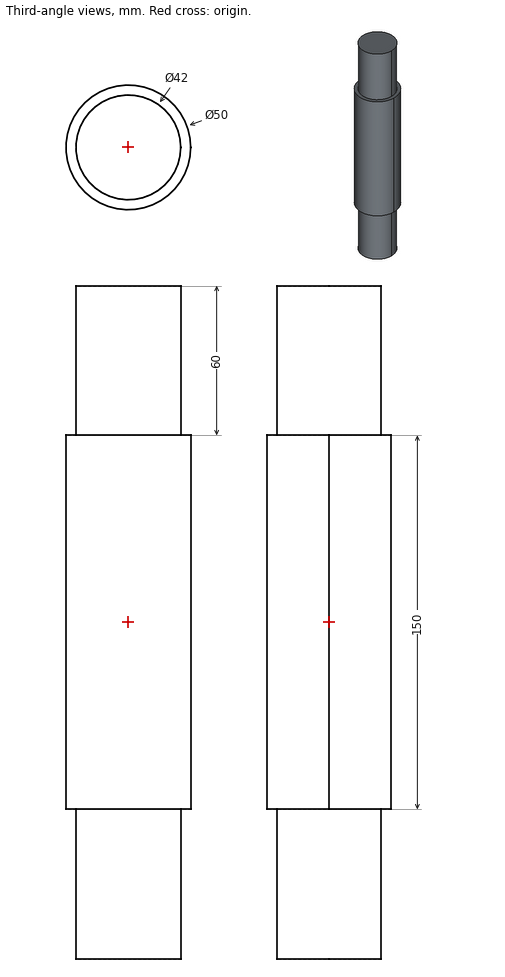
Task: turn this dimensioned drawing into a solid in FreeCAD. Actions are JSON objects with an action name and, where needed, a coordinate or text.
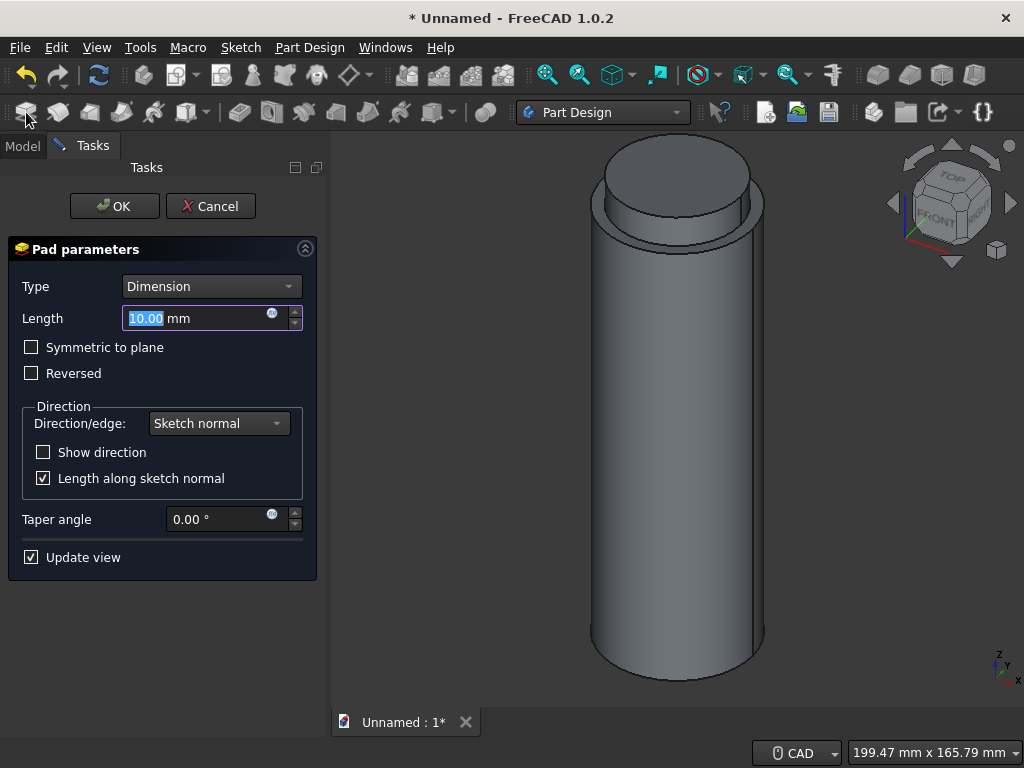
{"action": "type", "text": "60"}
{"action": "key", "text": "Tab"}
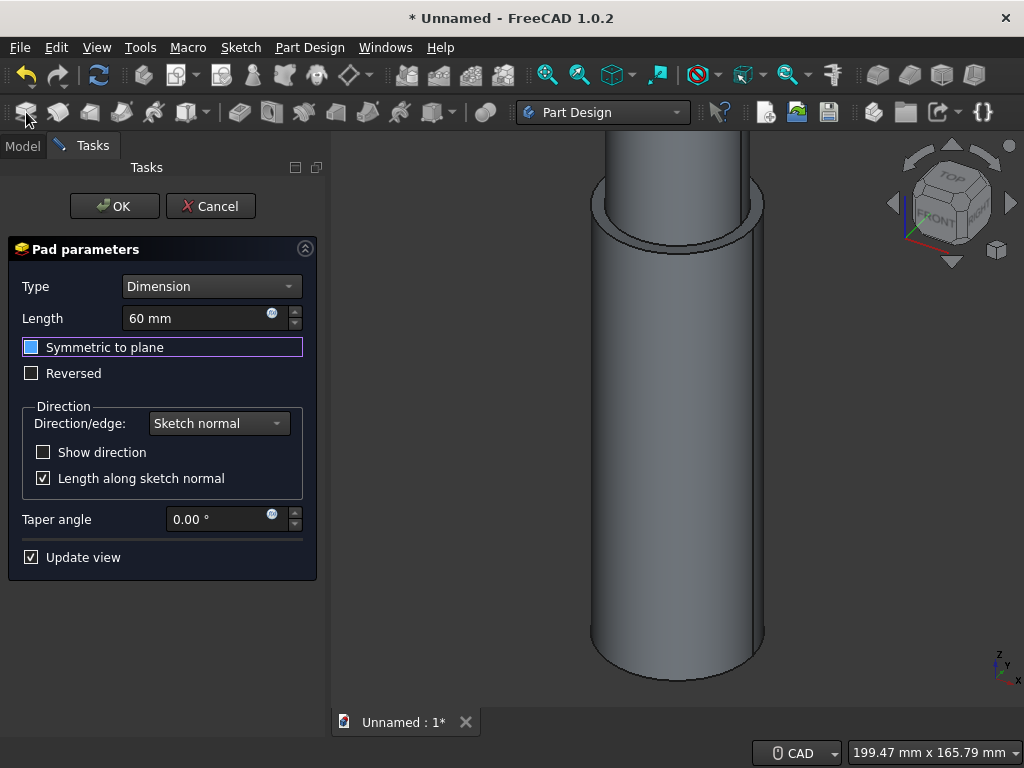
{"action": "left_click", "coordinate": [115, 206]}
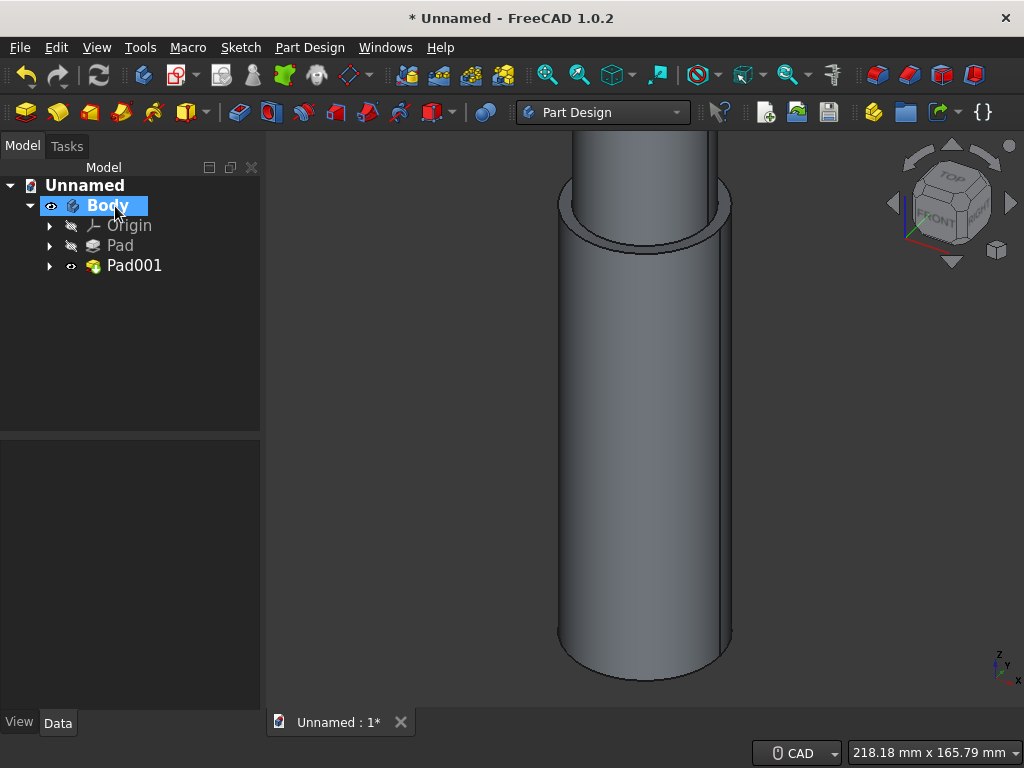
{"action": "left_click", "coordinate": [548, 76]}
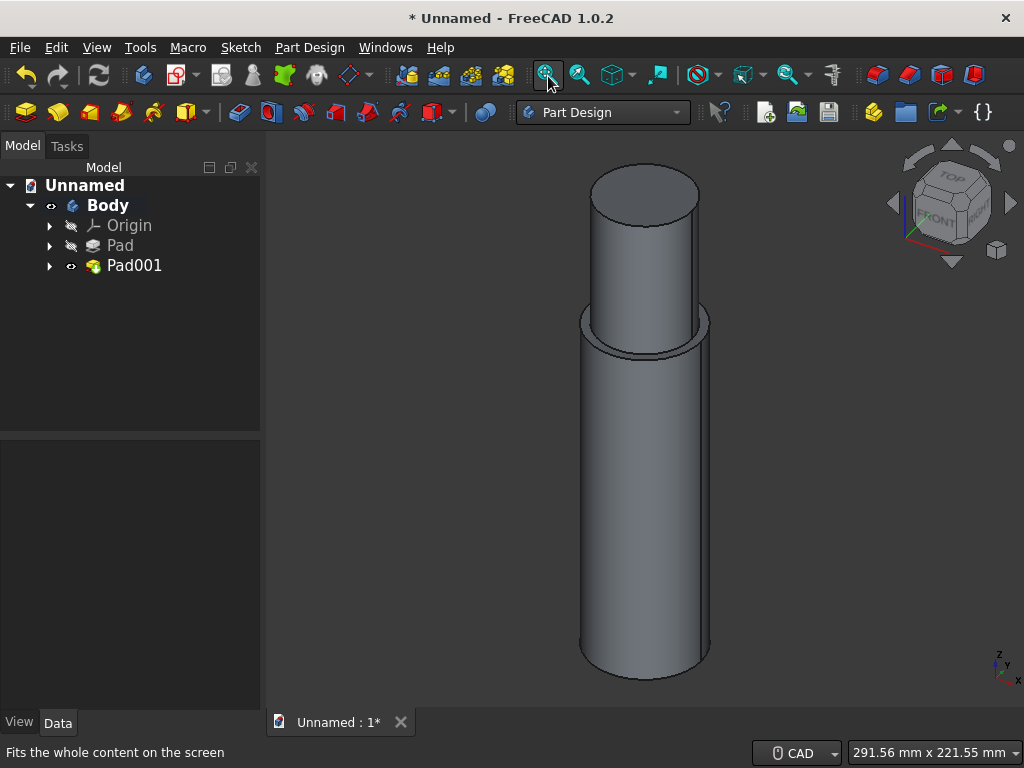
{"action": "left_click", "coordinate": [116, 266]}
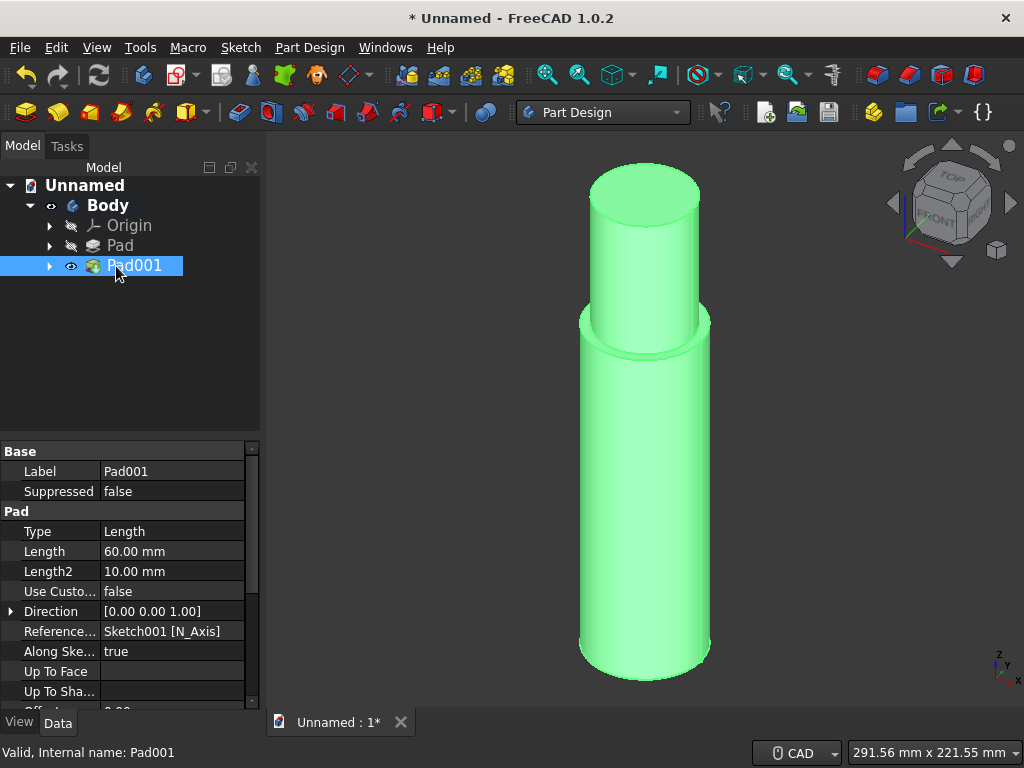
{"action": "left_click", "coordinate": [408, 76]}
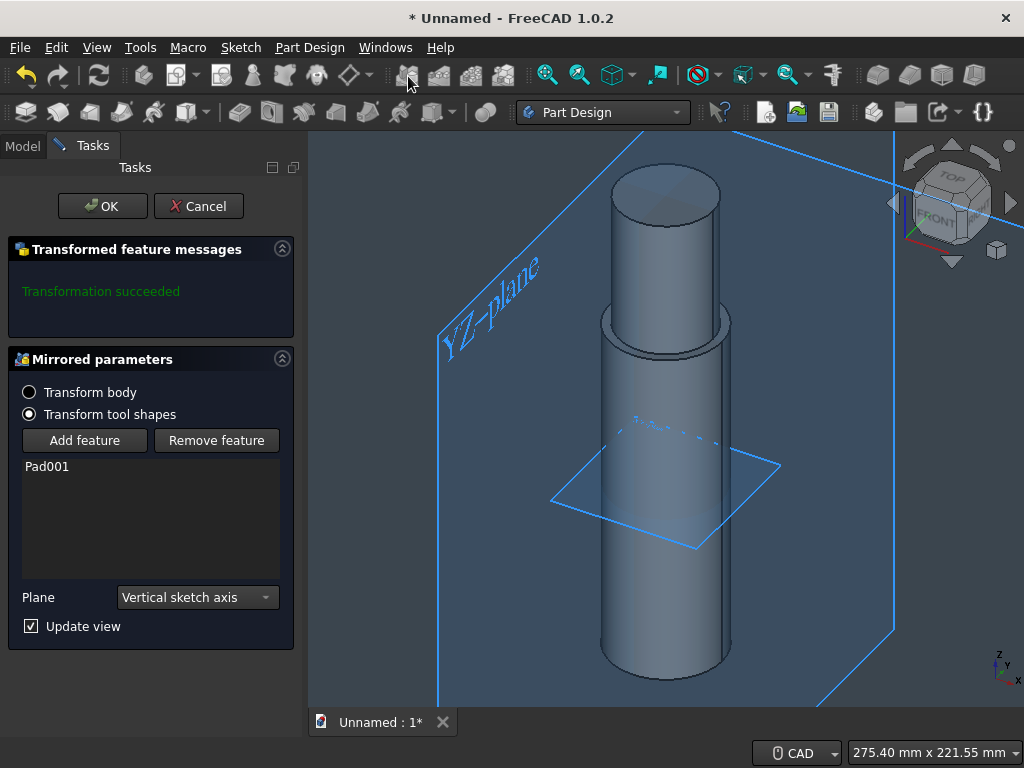
{"action": "left_click", "coordinate": [198, 598]}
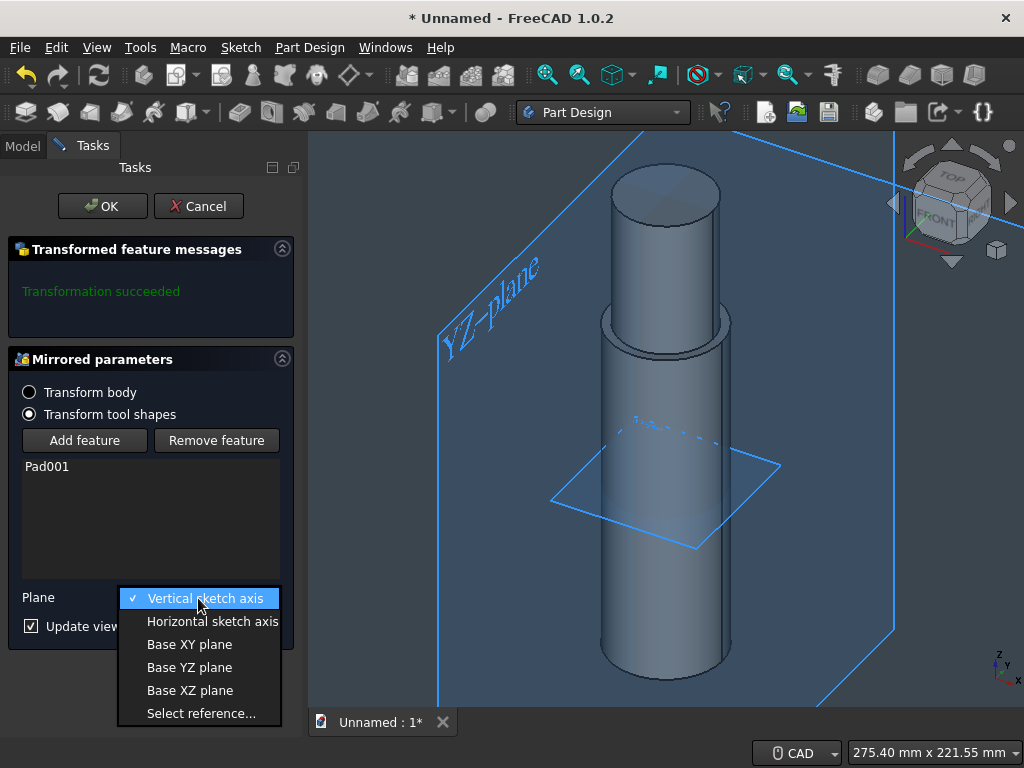
{"action": "left_click", "coordinate": [198, 644]}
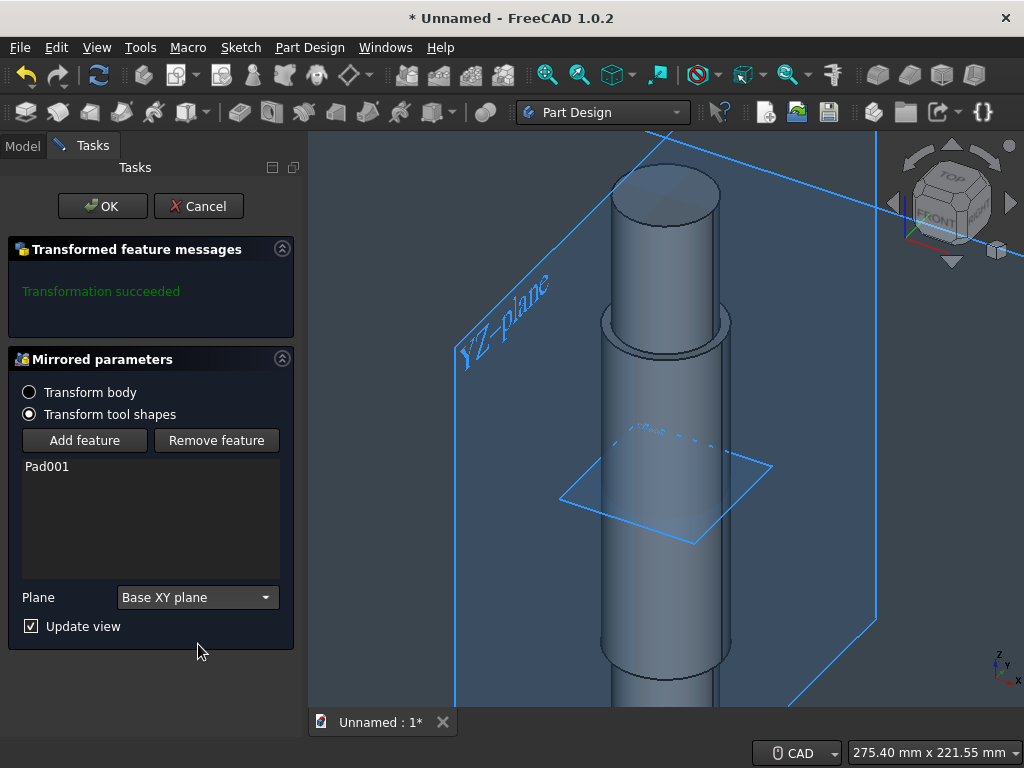
{"action": "left_click", "coordinate": [103, 206]}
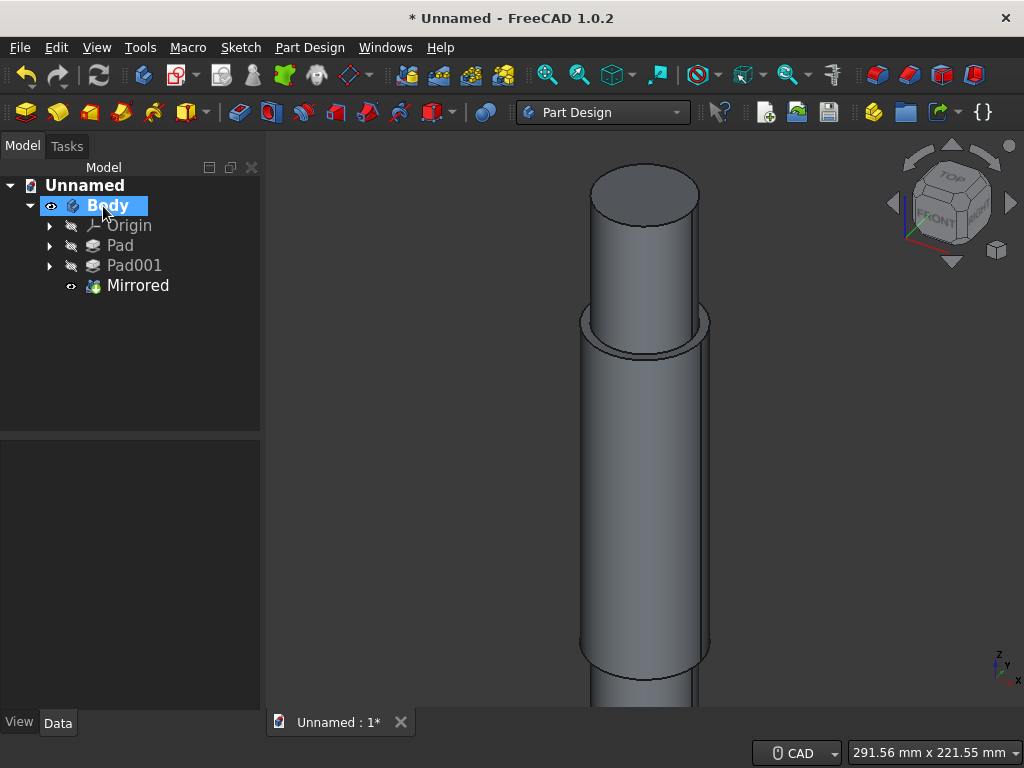
{"action": "key", "text": "0"}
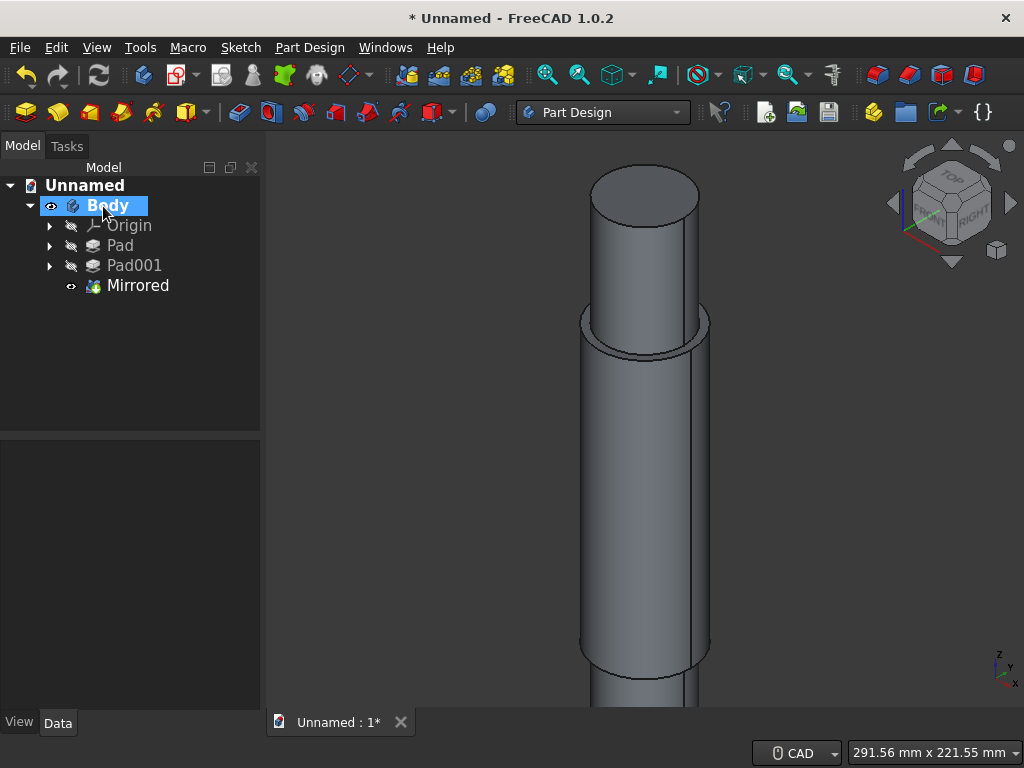
{"action": "left_click", "coordinate": [548, 76]}